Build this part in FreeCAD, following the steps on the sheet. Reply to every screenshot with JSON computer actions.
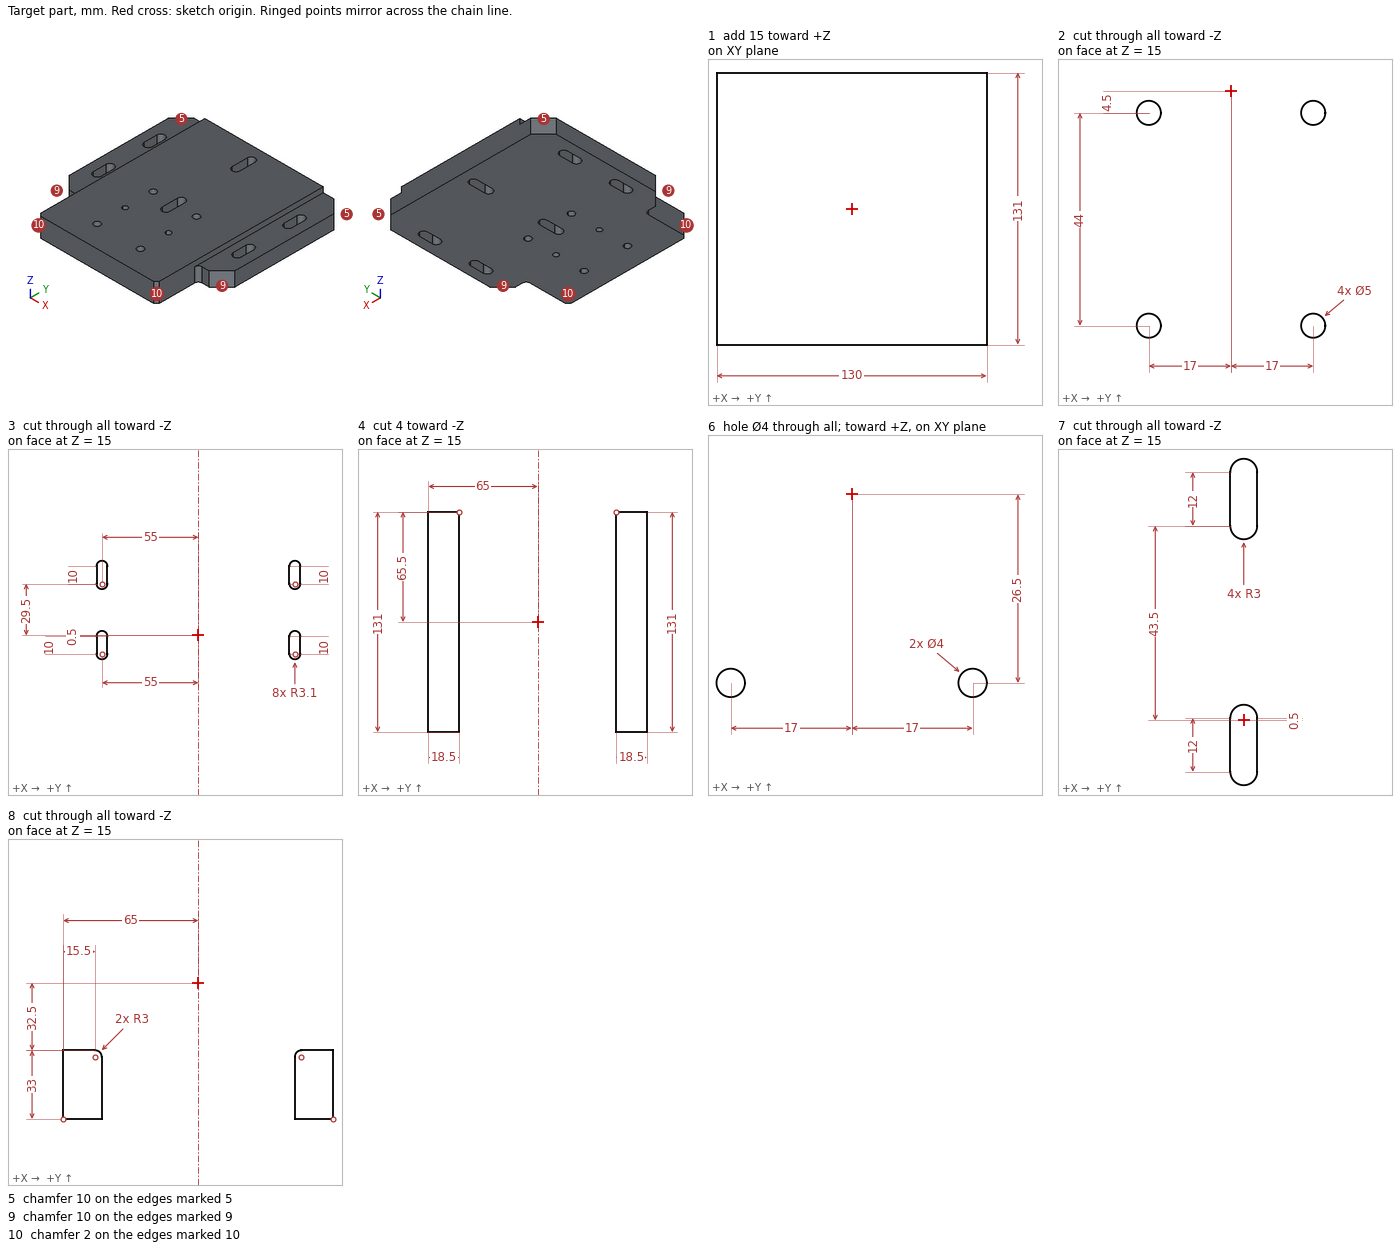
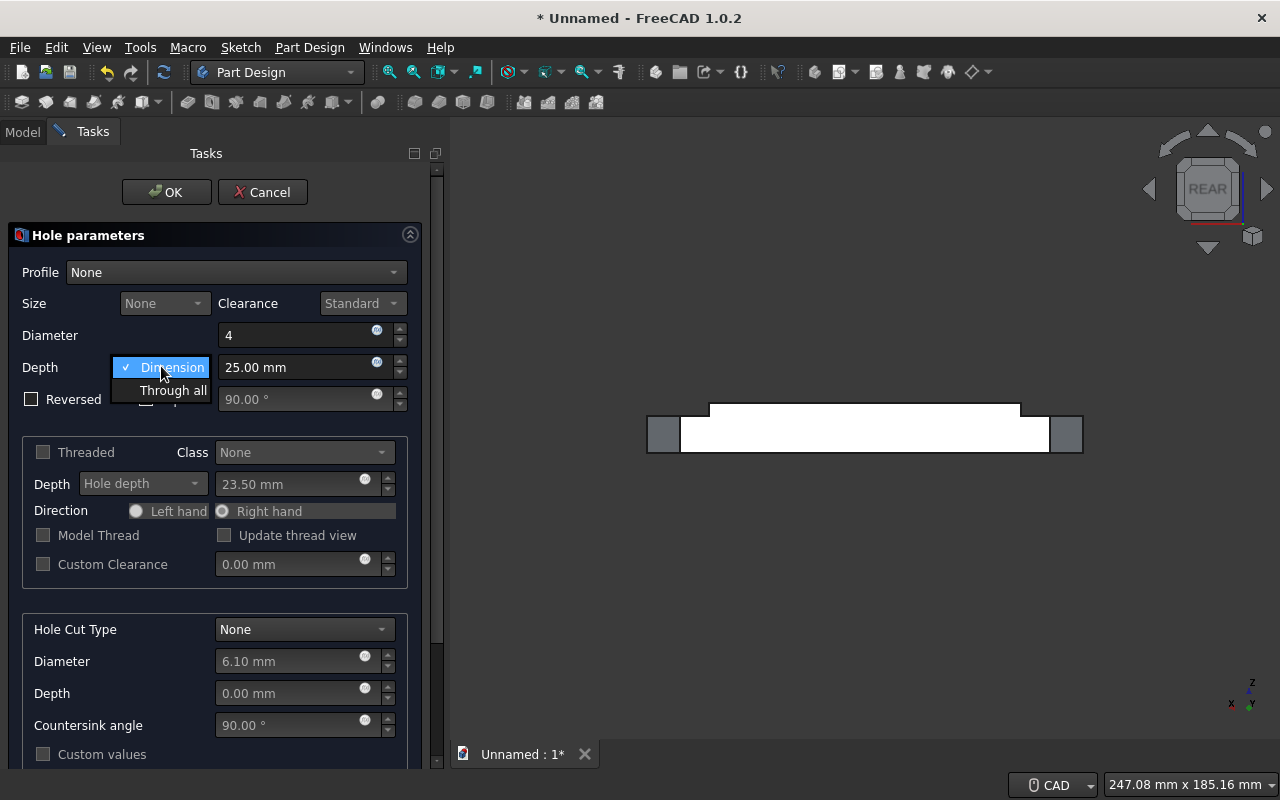
{"action": "left_click", "coordinate": [160, 390]}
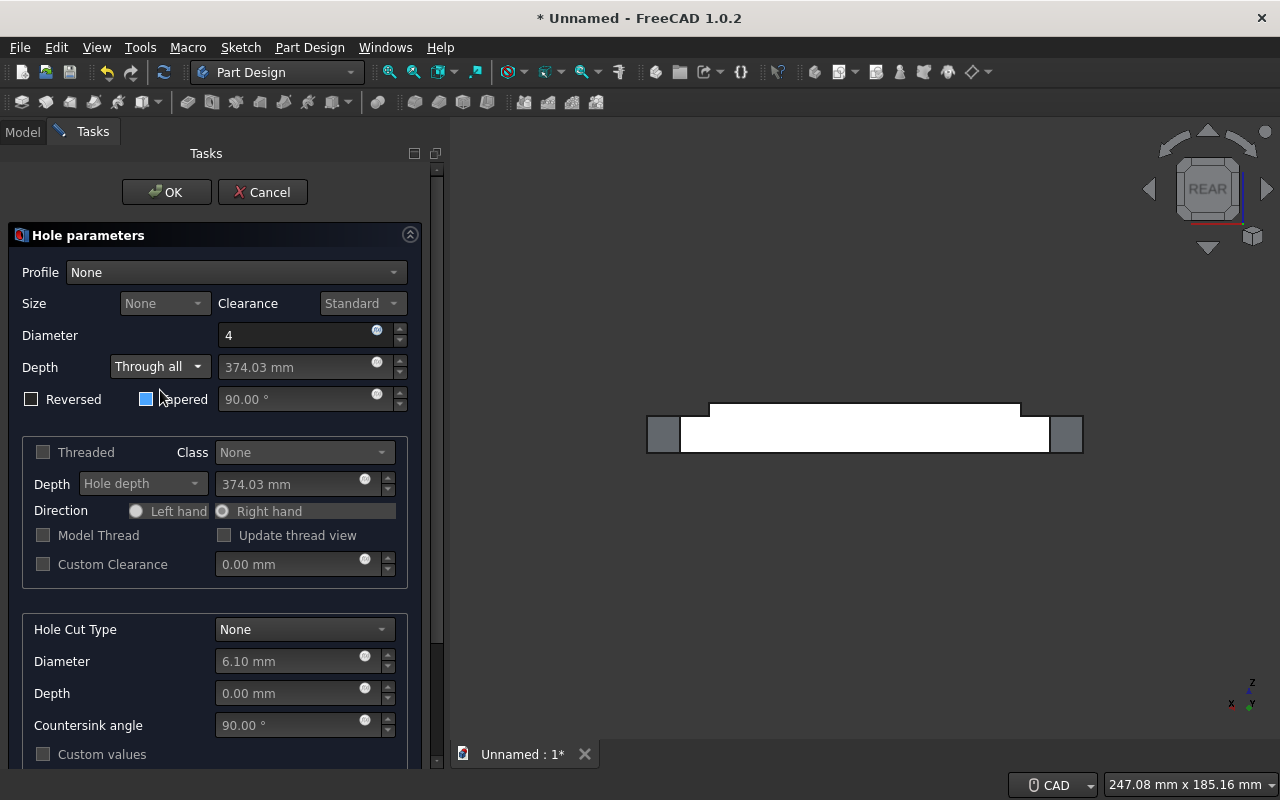
{"action": "left_click", "coordinate": [30, 399]}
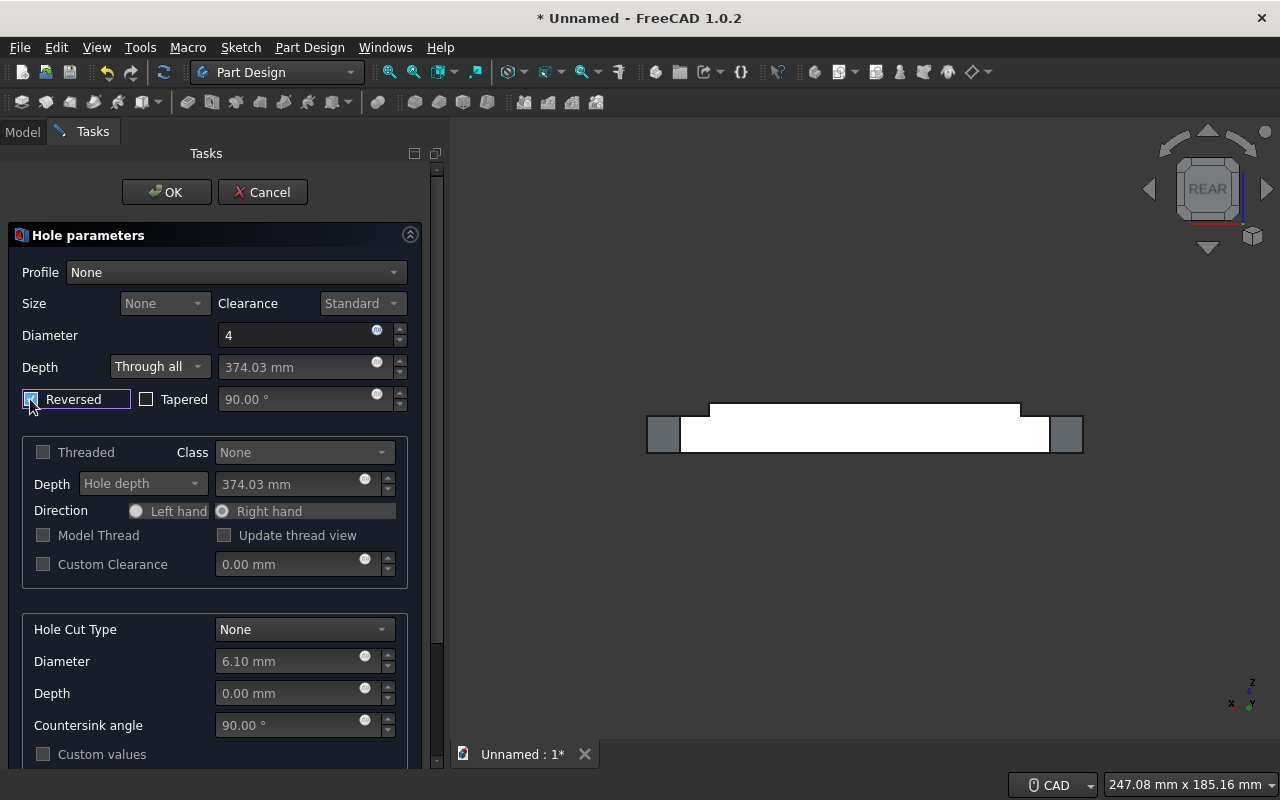
{"action": "left_click", "coordinate": [167, 192]}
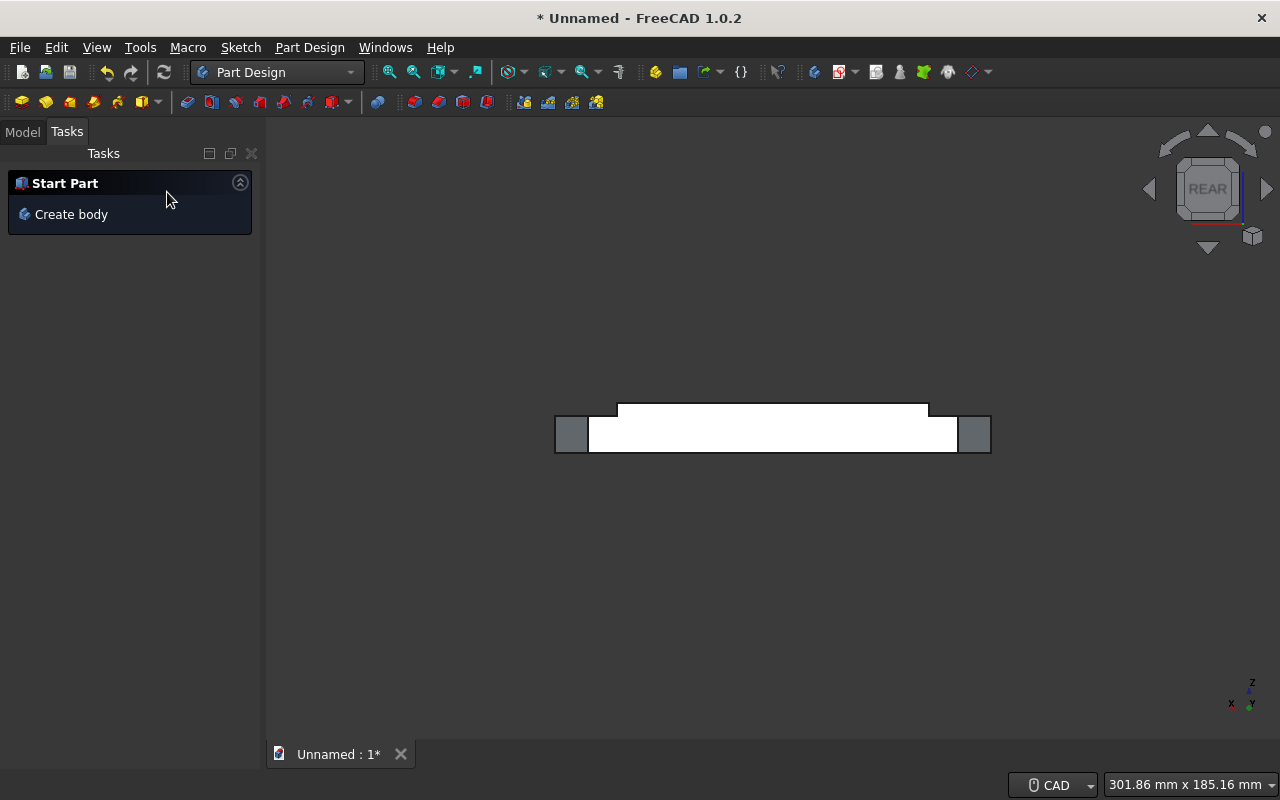
{"action": "key", "text": "v f"}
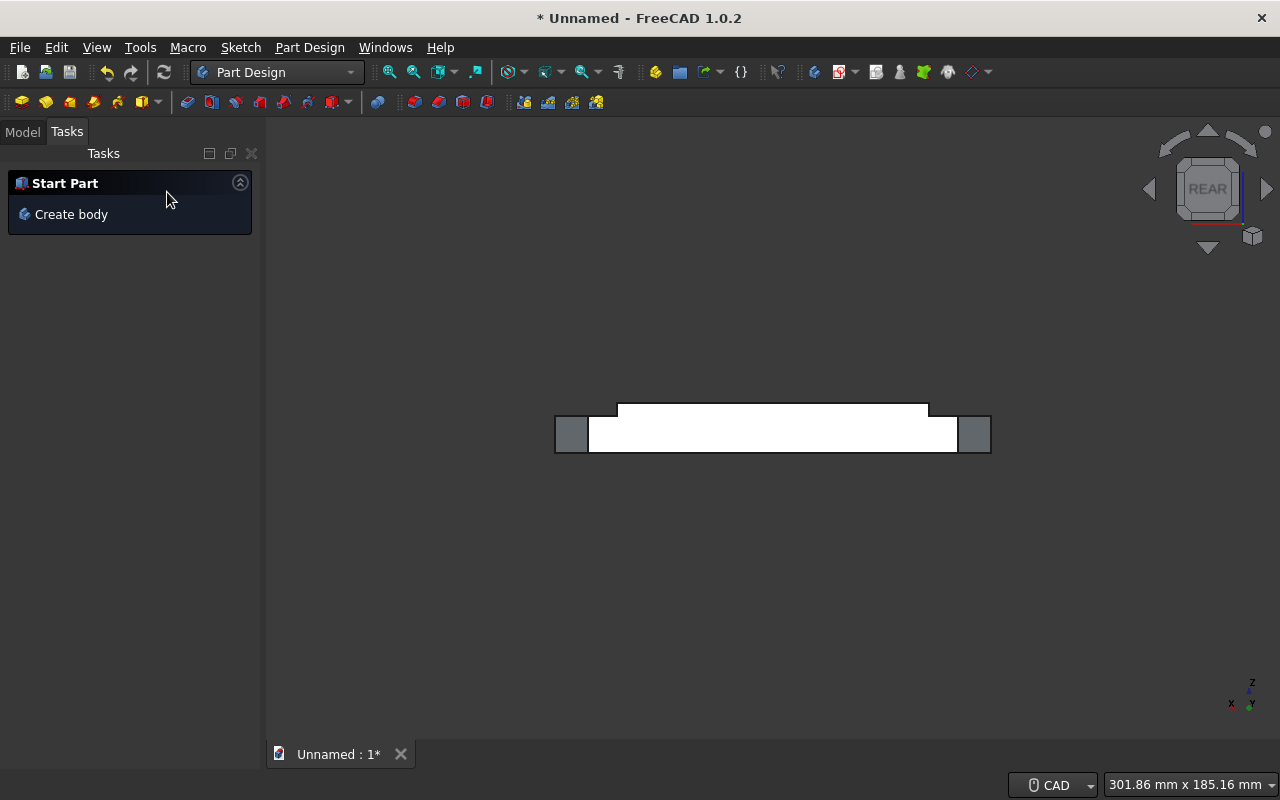
{"action": "key", "text": "0"}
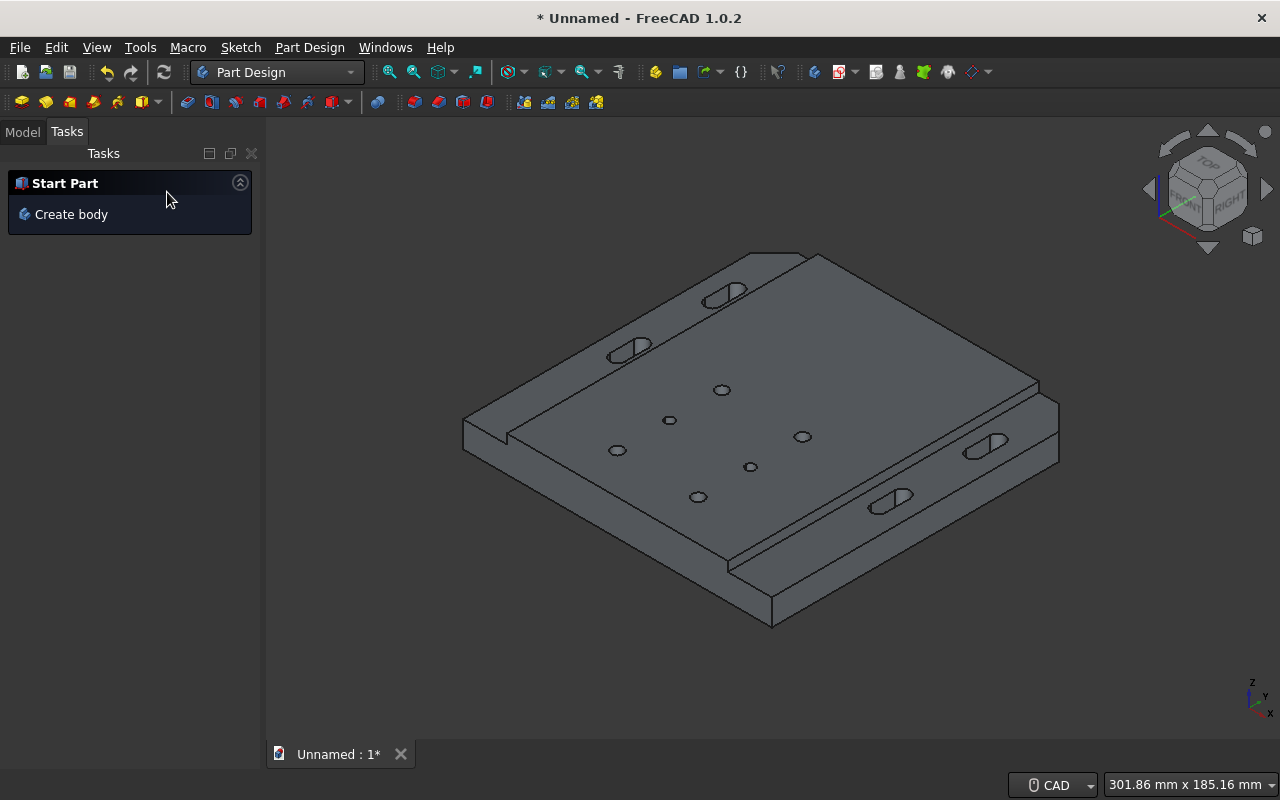
{"action": "left_click", "coordinate": [893, 373]}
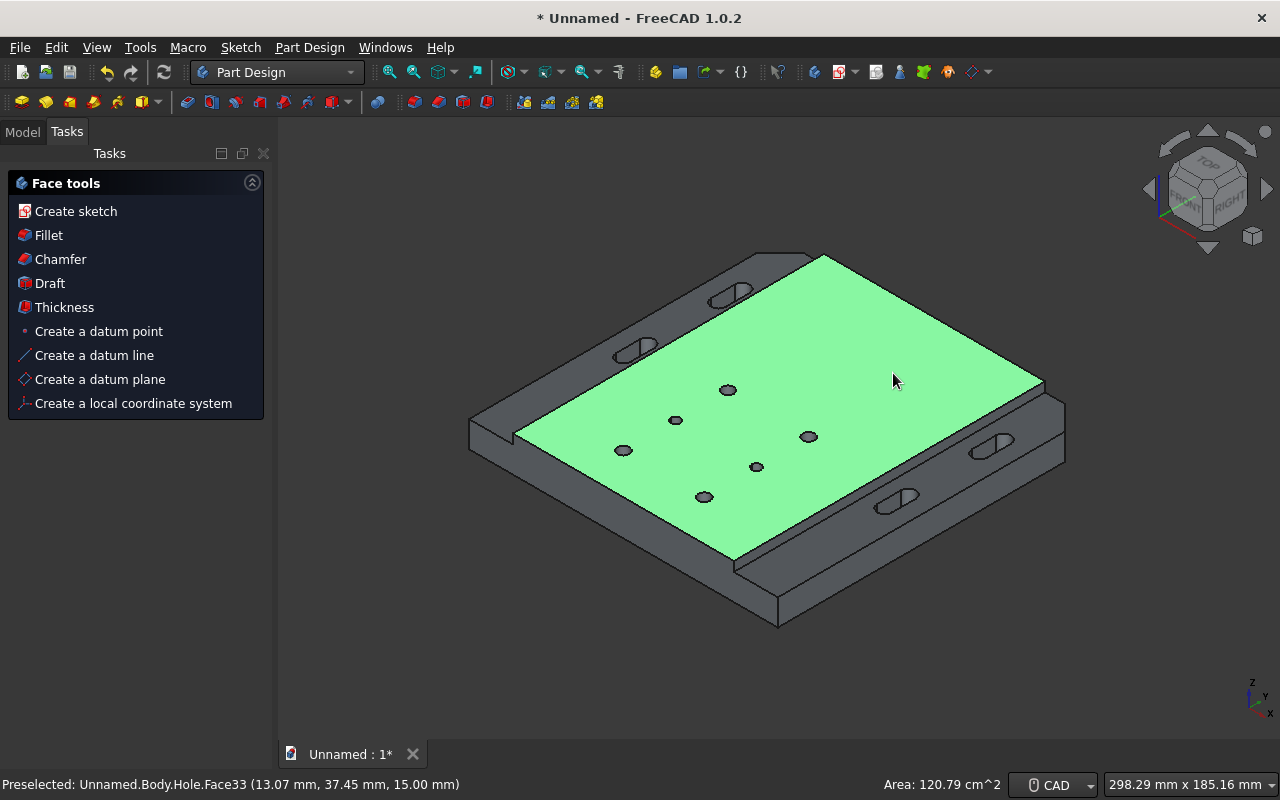
{"action": "left_click", "coordinate": [840, 72]}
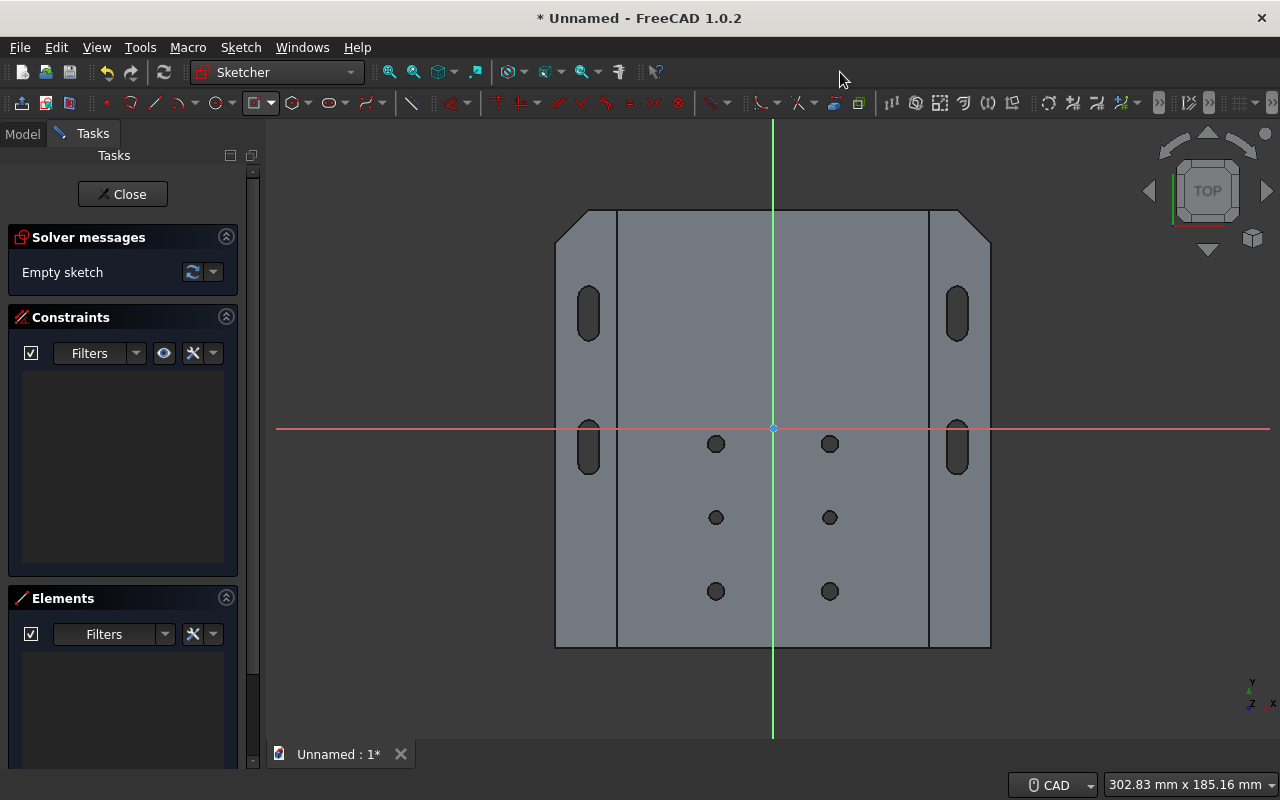
{"action": "scroll", "coordinate": [912, 206], "scroll_direction": "up", "scroll_amount": 2}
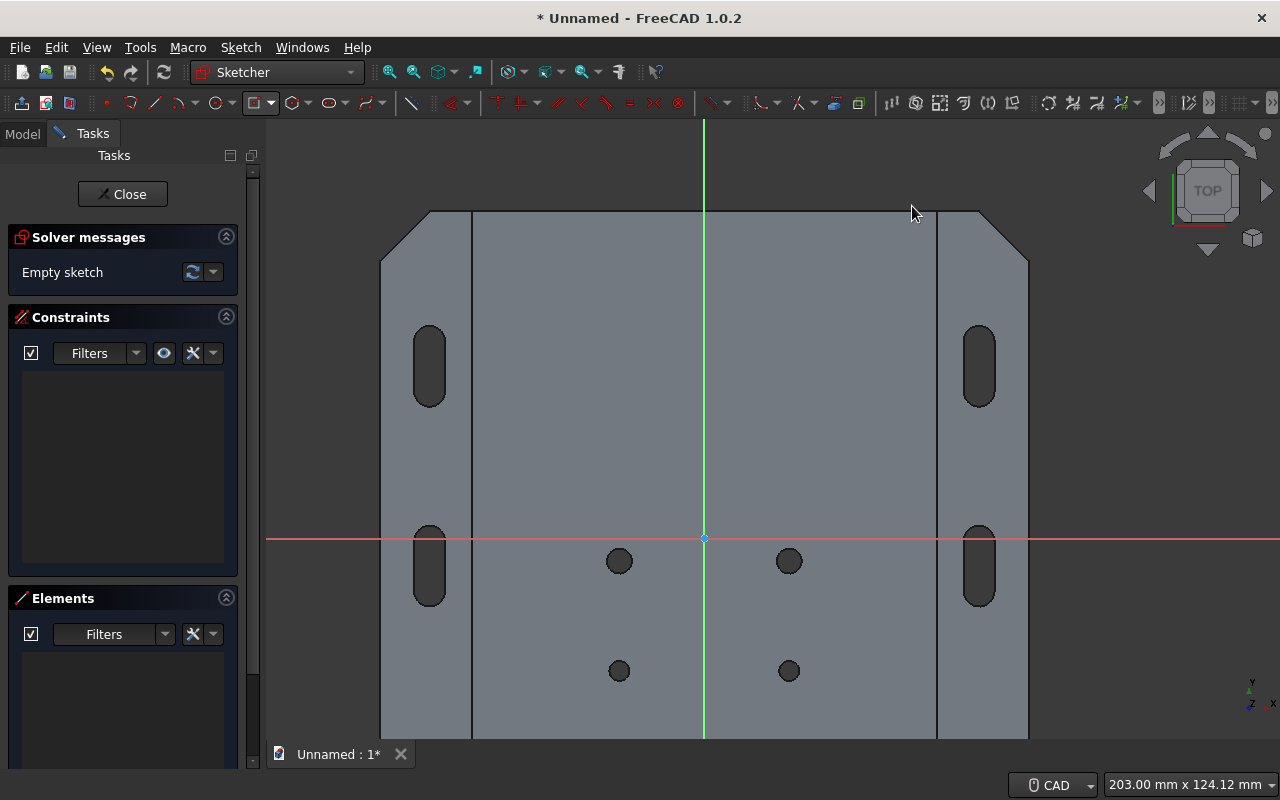
{"action": "left_click", "coordinate": [330, 104]}